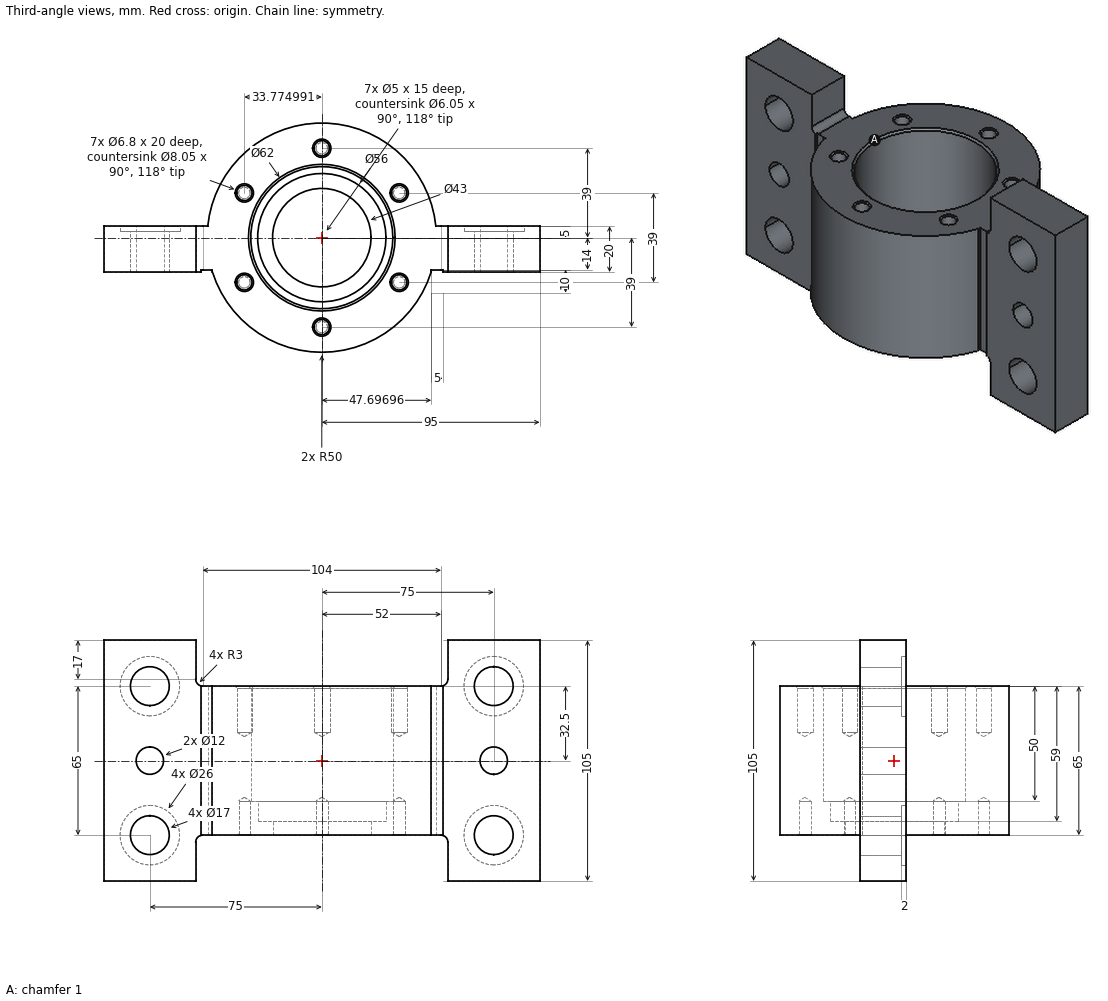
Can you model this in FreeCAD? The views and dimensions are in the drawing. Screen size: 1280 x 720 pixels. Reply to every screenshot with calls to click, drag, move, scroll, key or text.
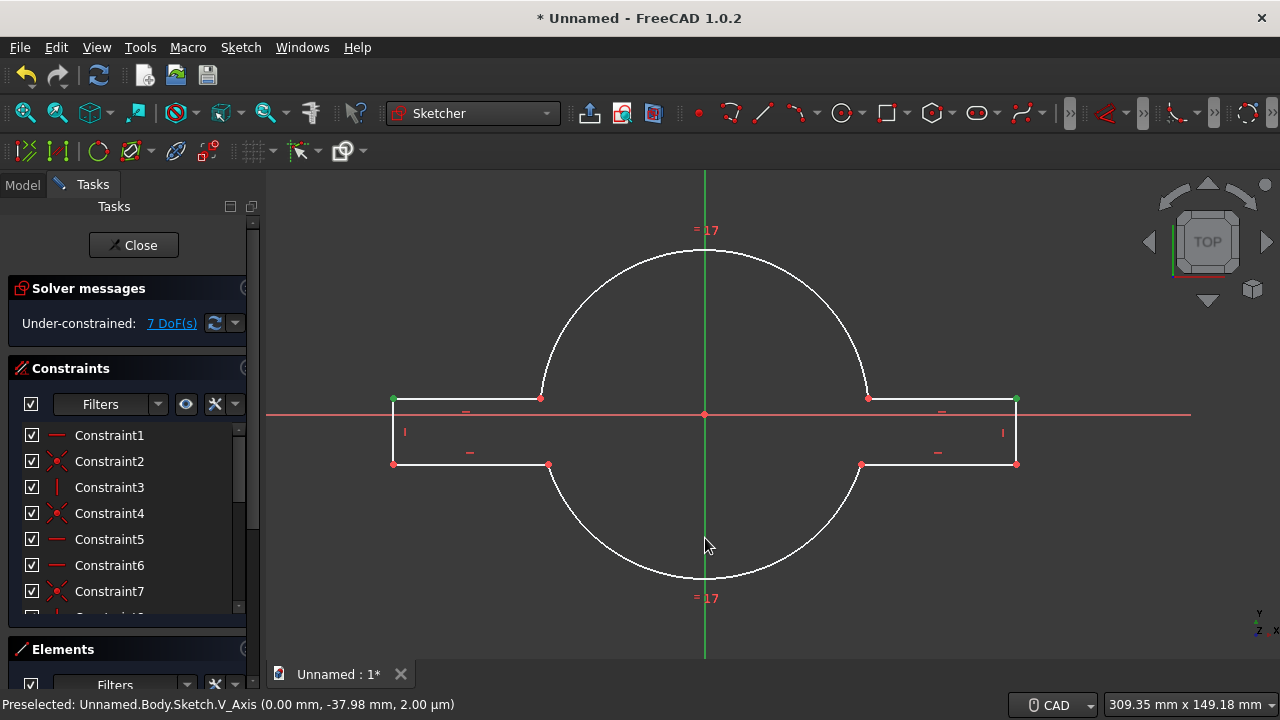
key(s)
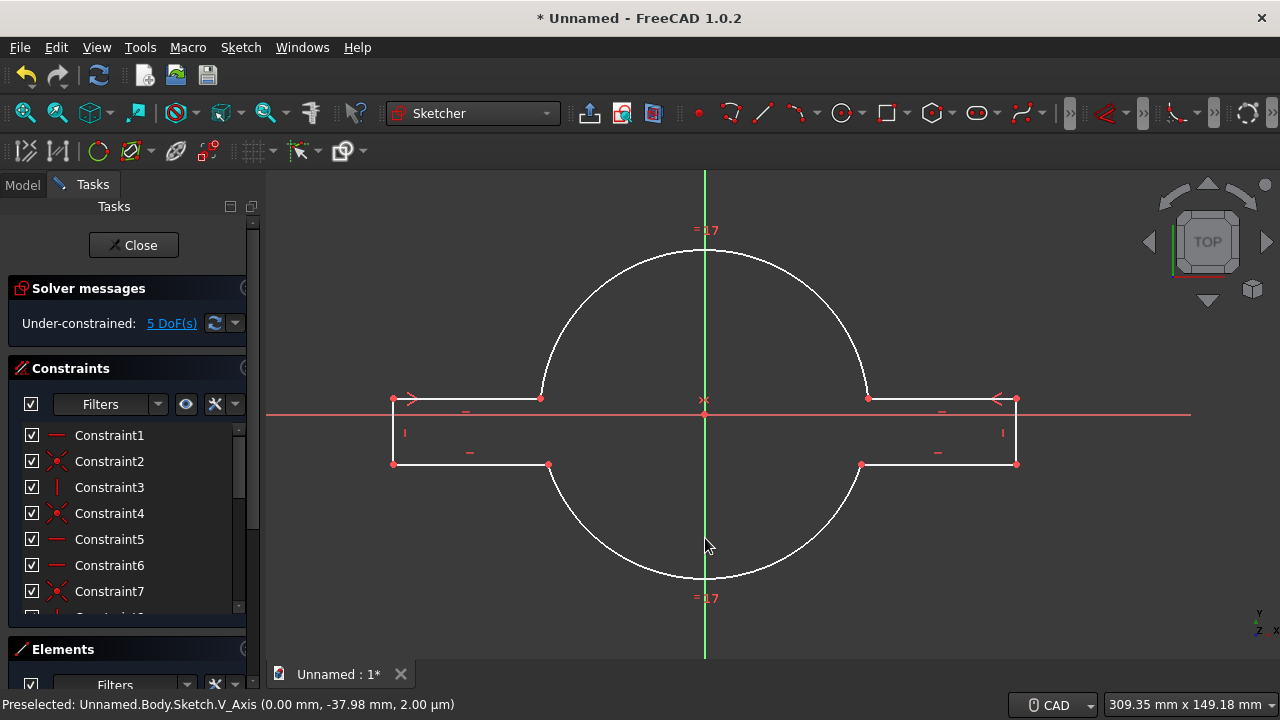
click(1106, 114)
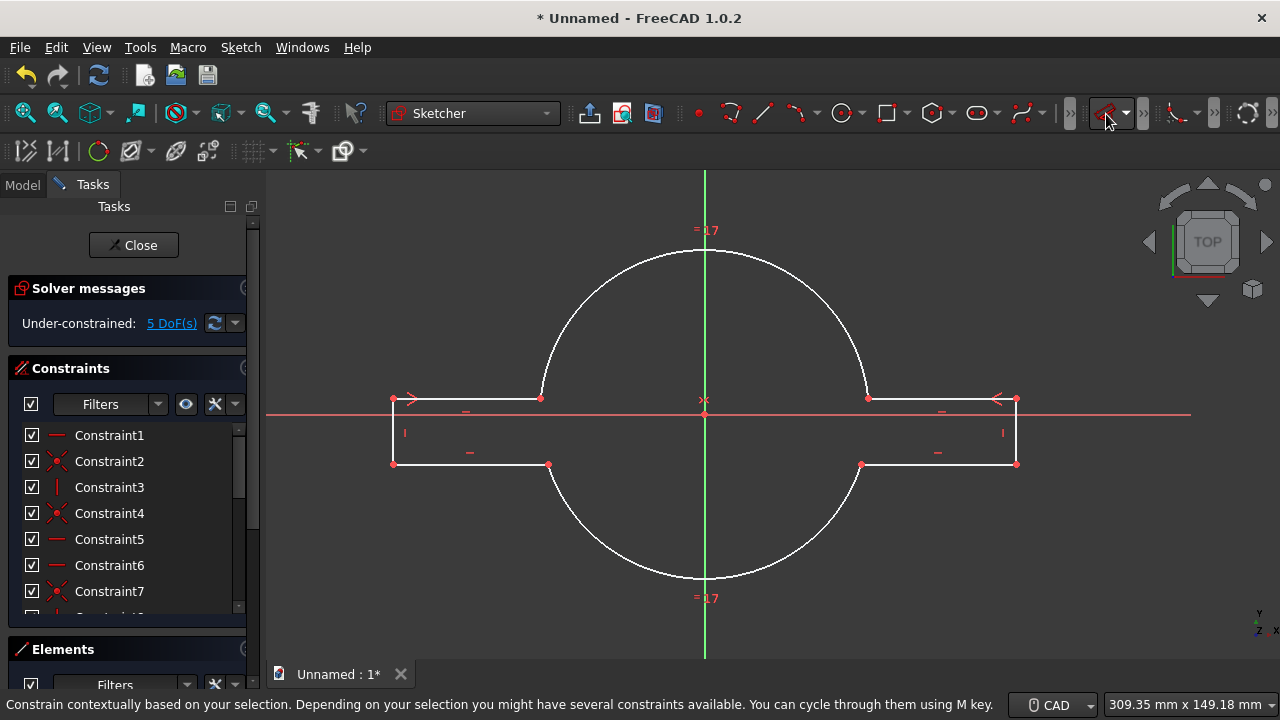
click(796, 278)
click(814, 251)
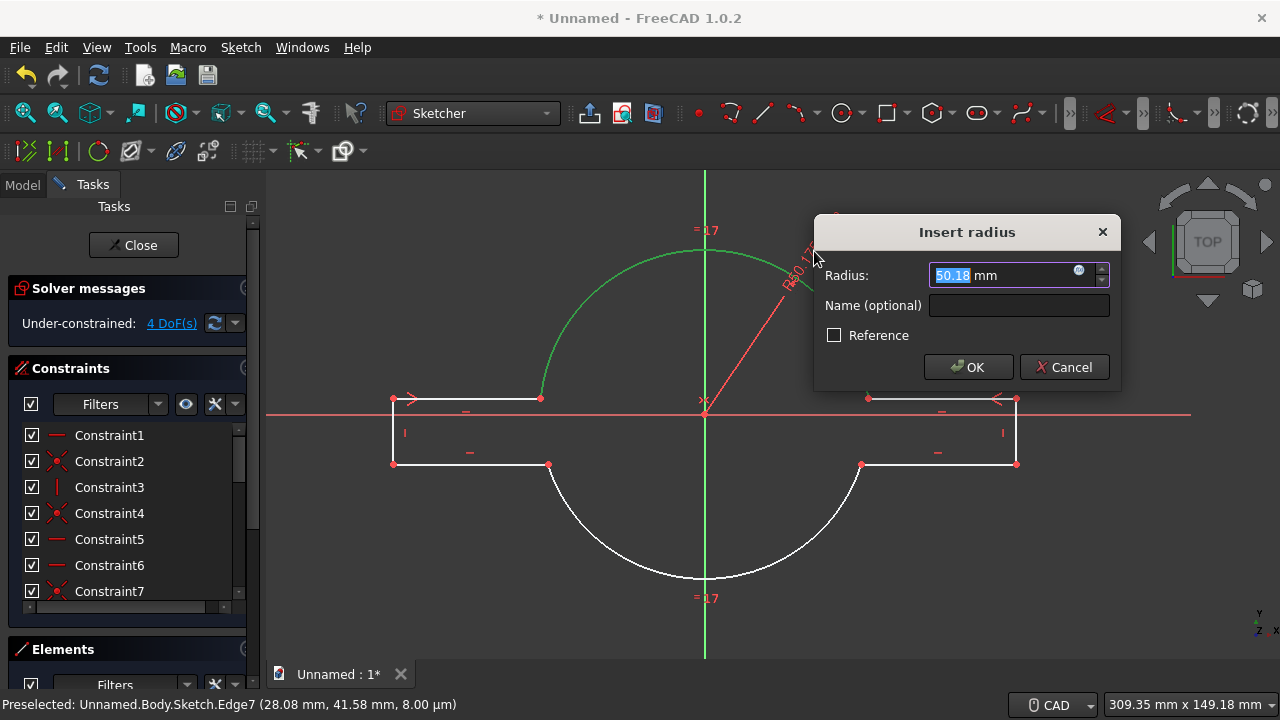
text(50)
key(Return)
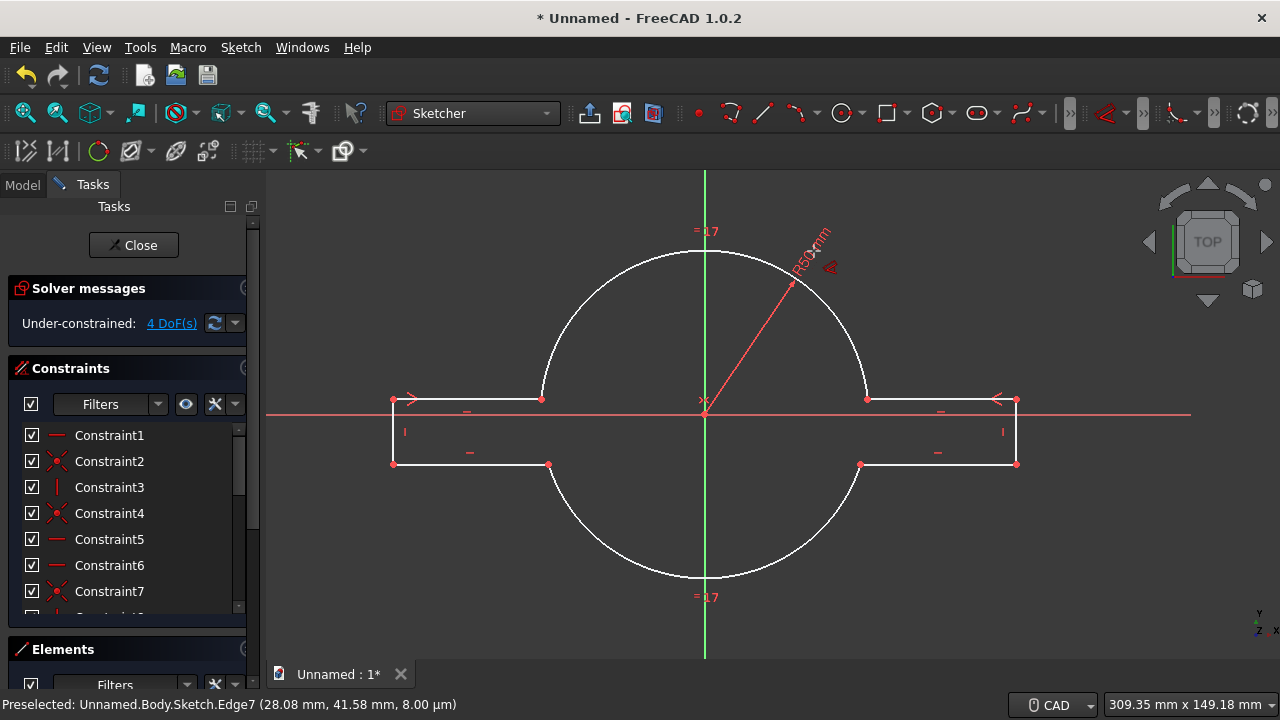
click(1016, 445)
click(1050, 432)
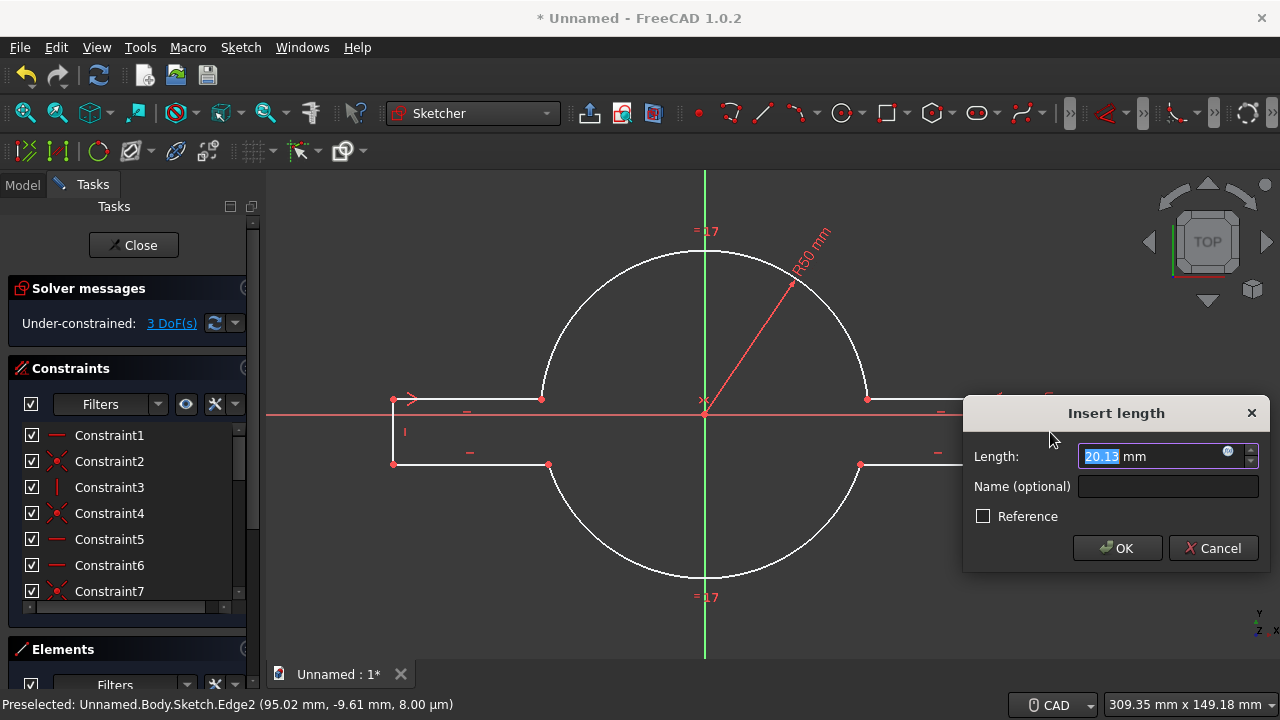
text(20)
key(Return)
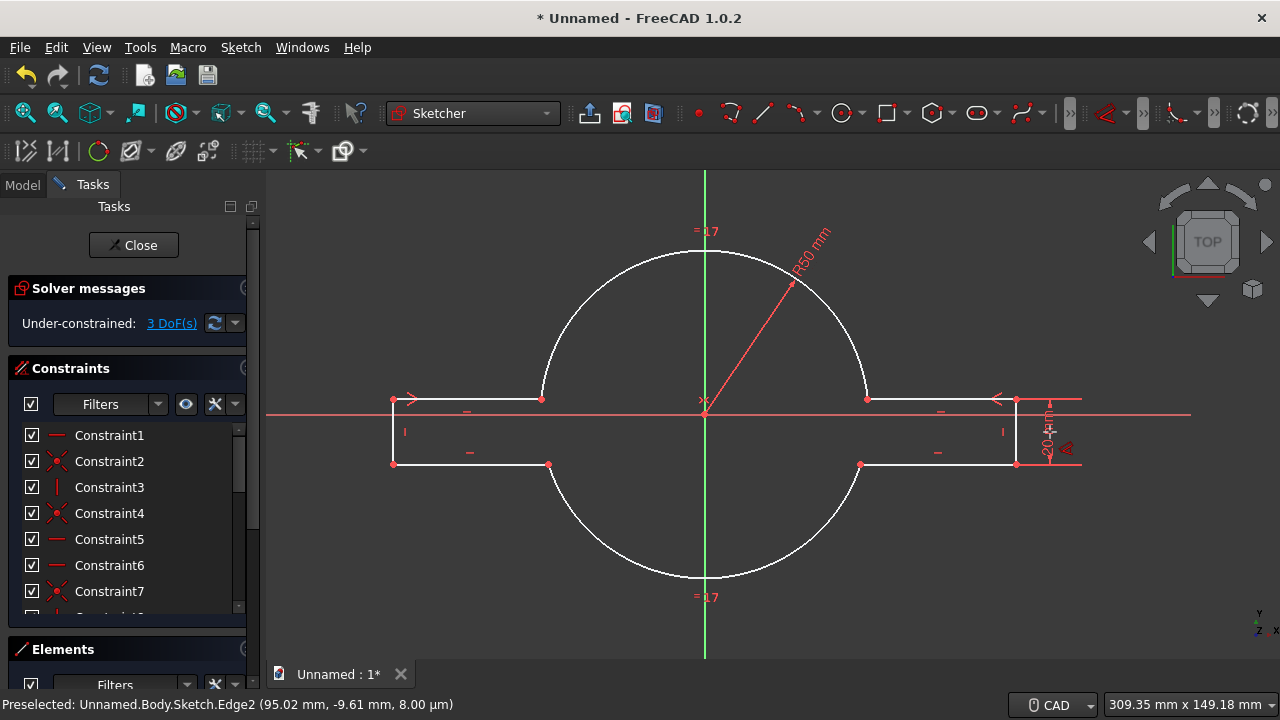
click(393, 445)
click(359, 432)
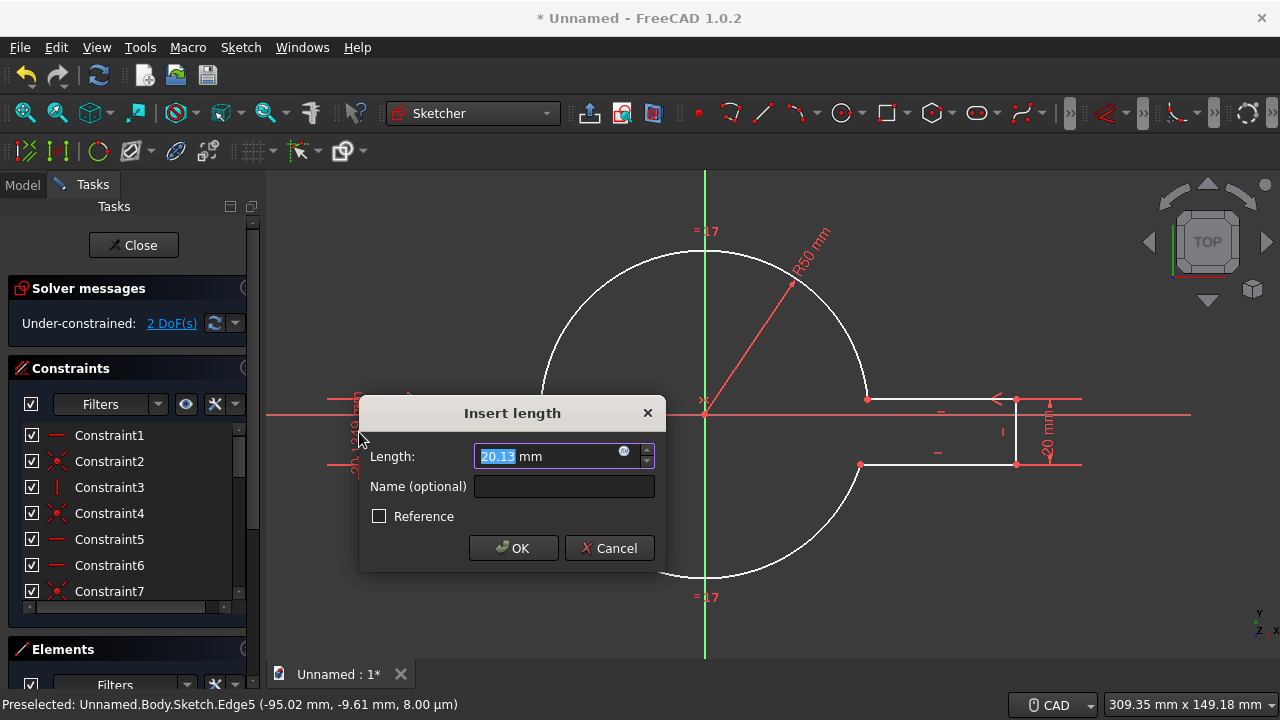
text(20)
key(Return)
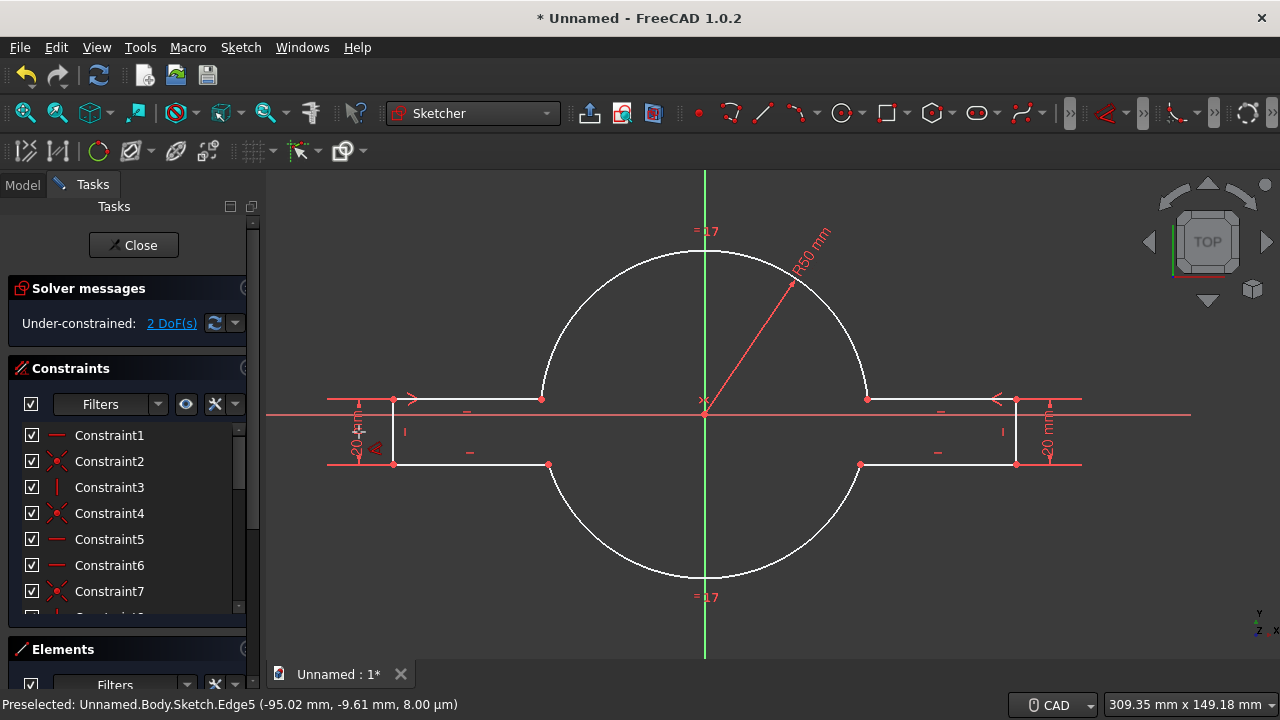
scroll(1016, 399, up, 5)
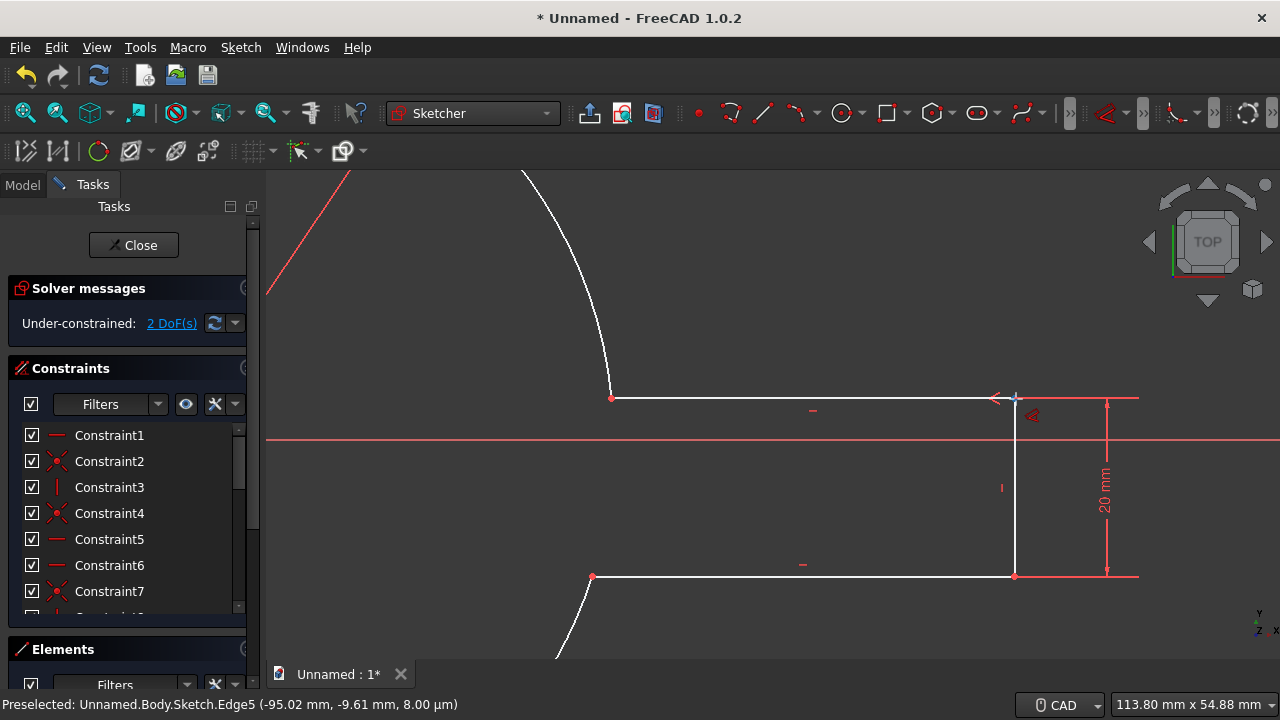
click(1015, 398)
click(1049, 419)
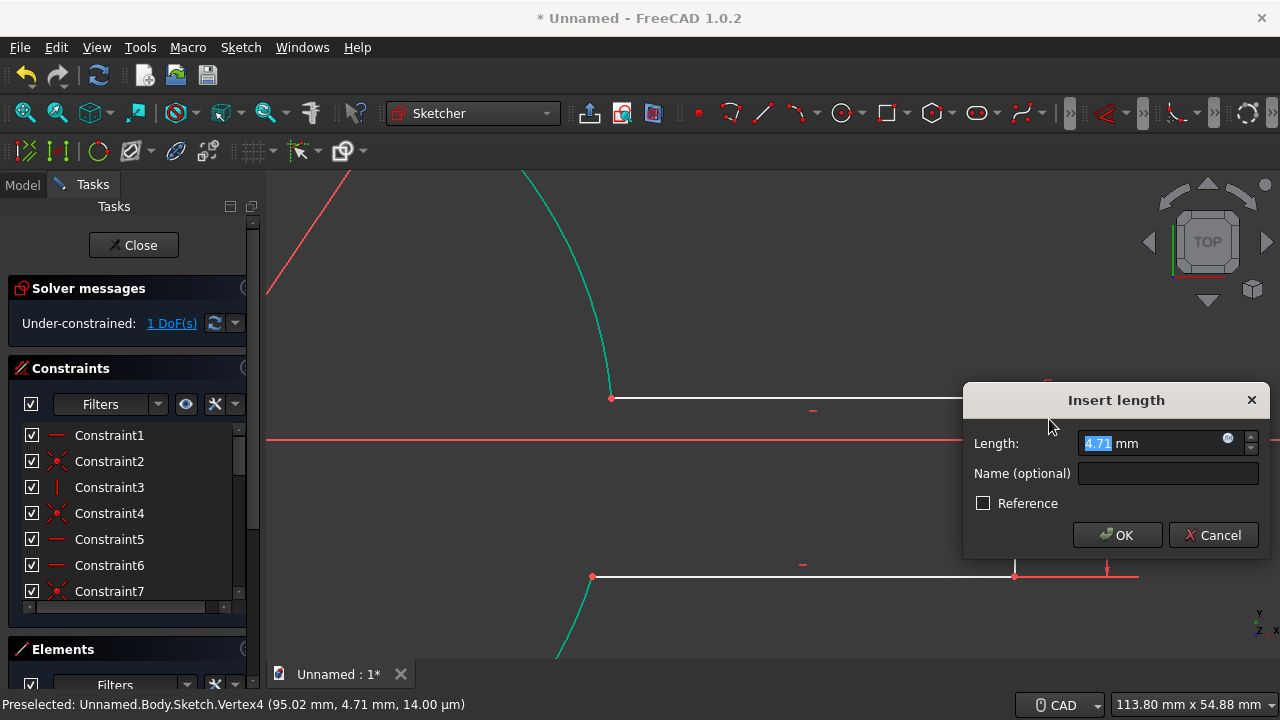
text(5)
key(Return)